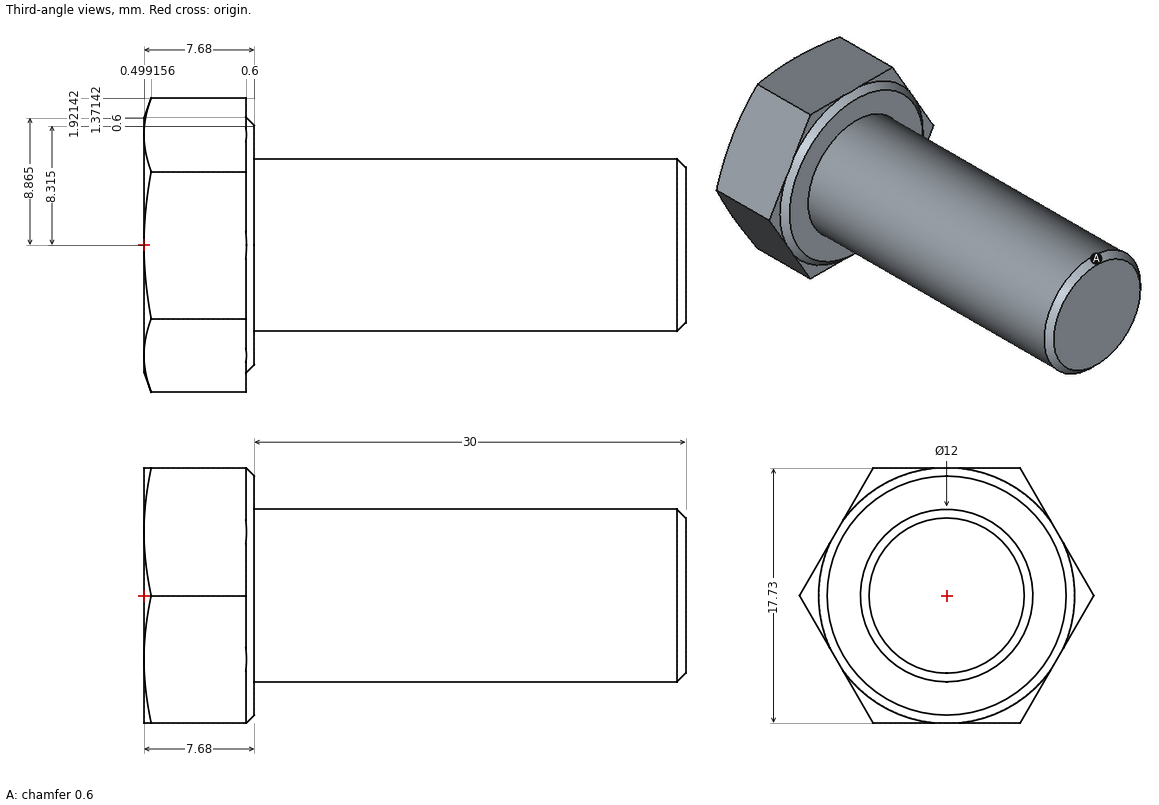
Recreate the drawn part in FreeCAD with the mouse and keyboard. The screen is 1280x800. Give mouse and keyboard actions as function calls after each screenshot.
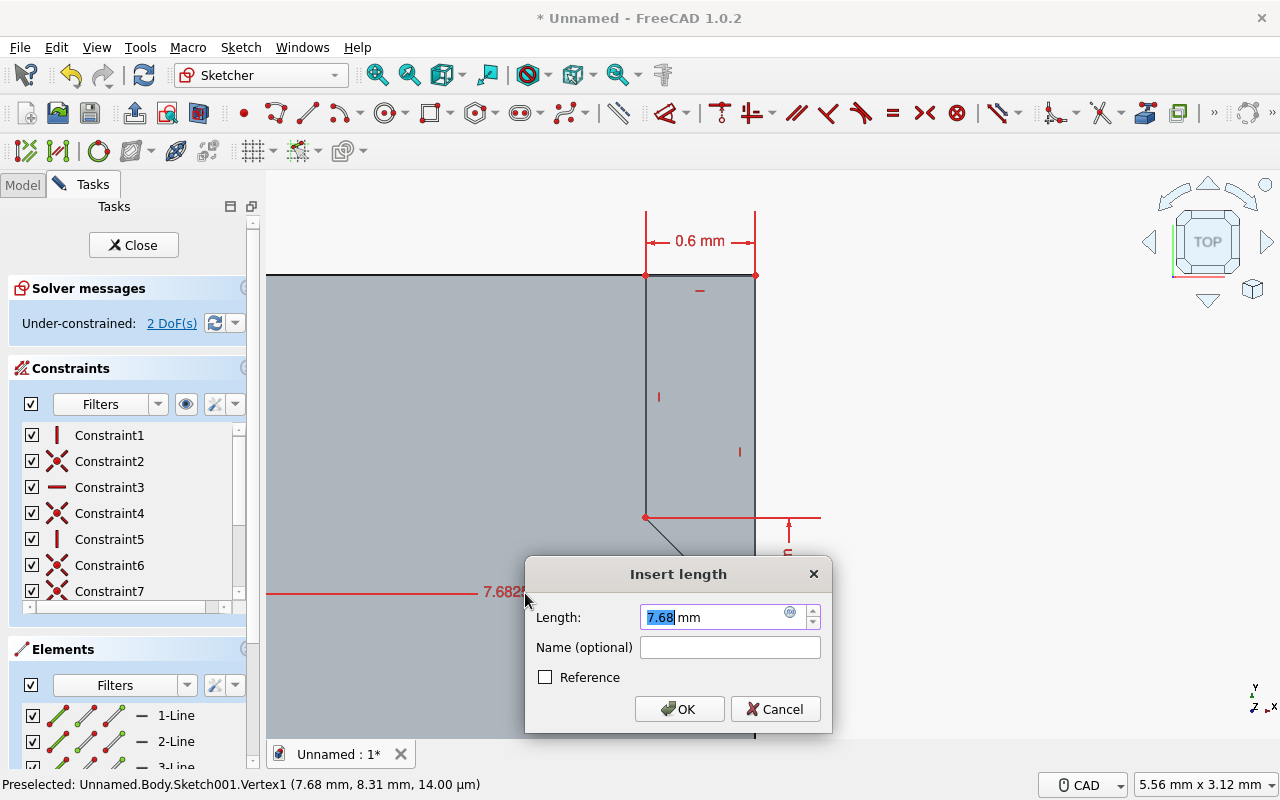
text(7.68)
key(Return)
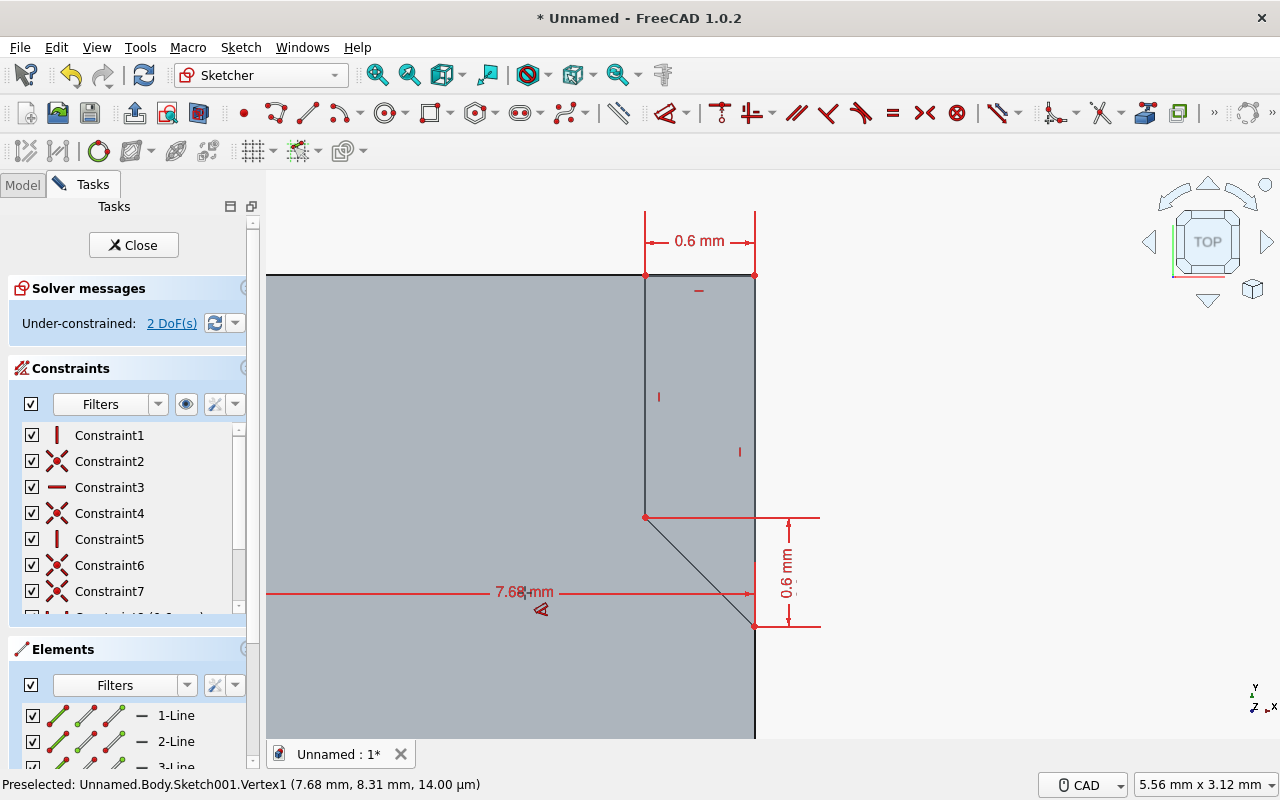
click(755, 627)
click(789, 669)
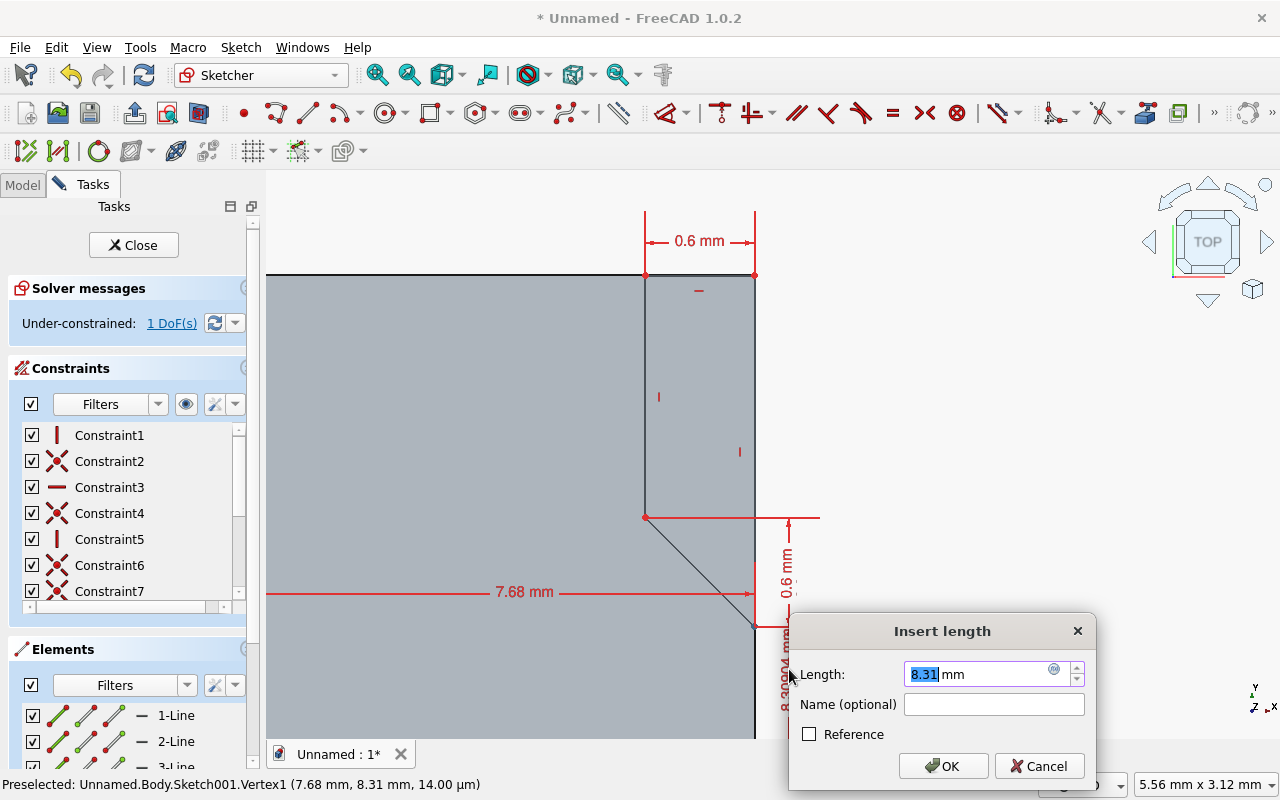
text(8.315)
key(Return)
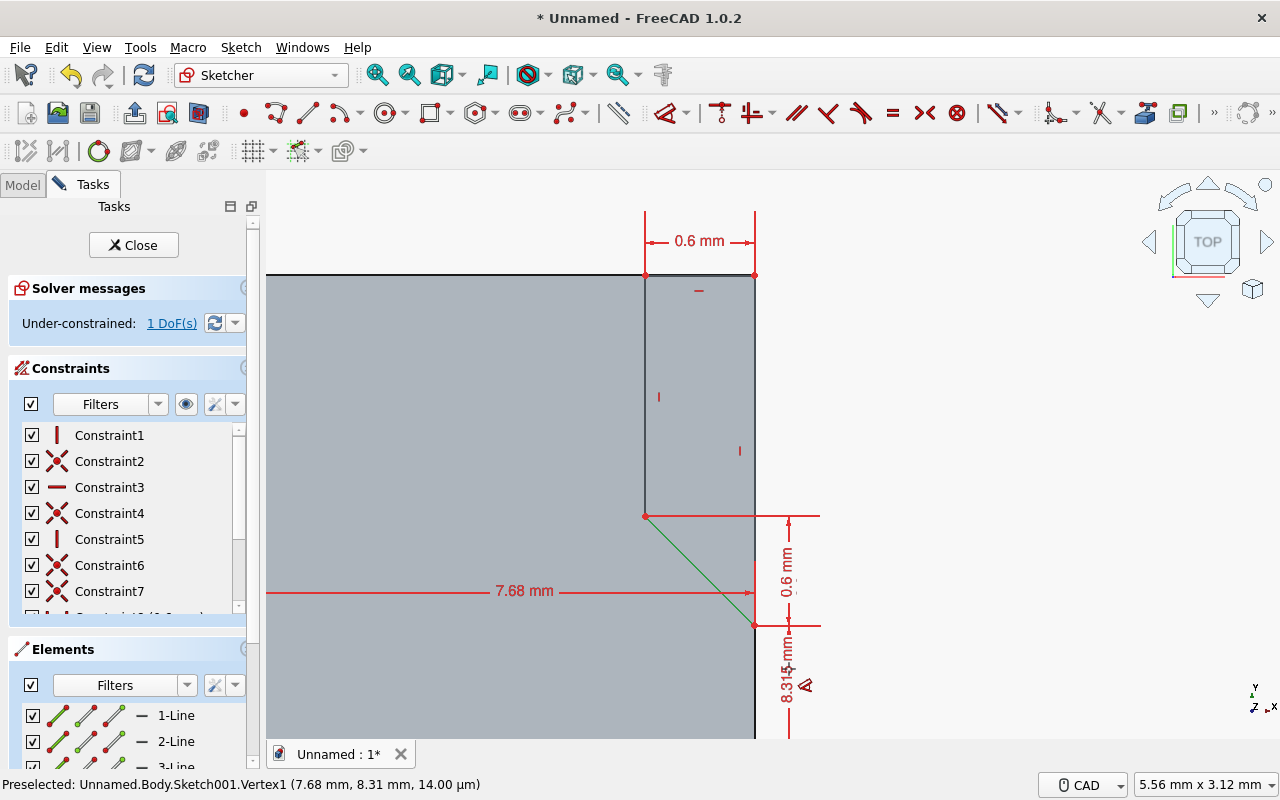
click(755, 521)
click(789, 451)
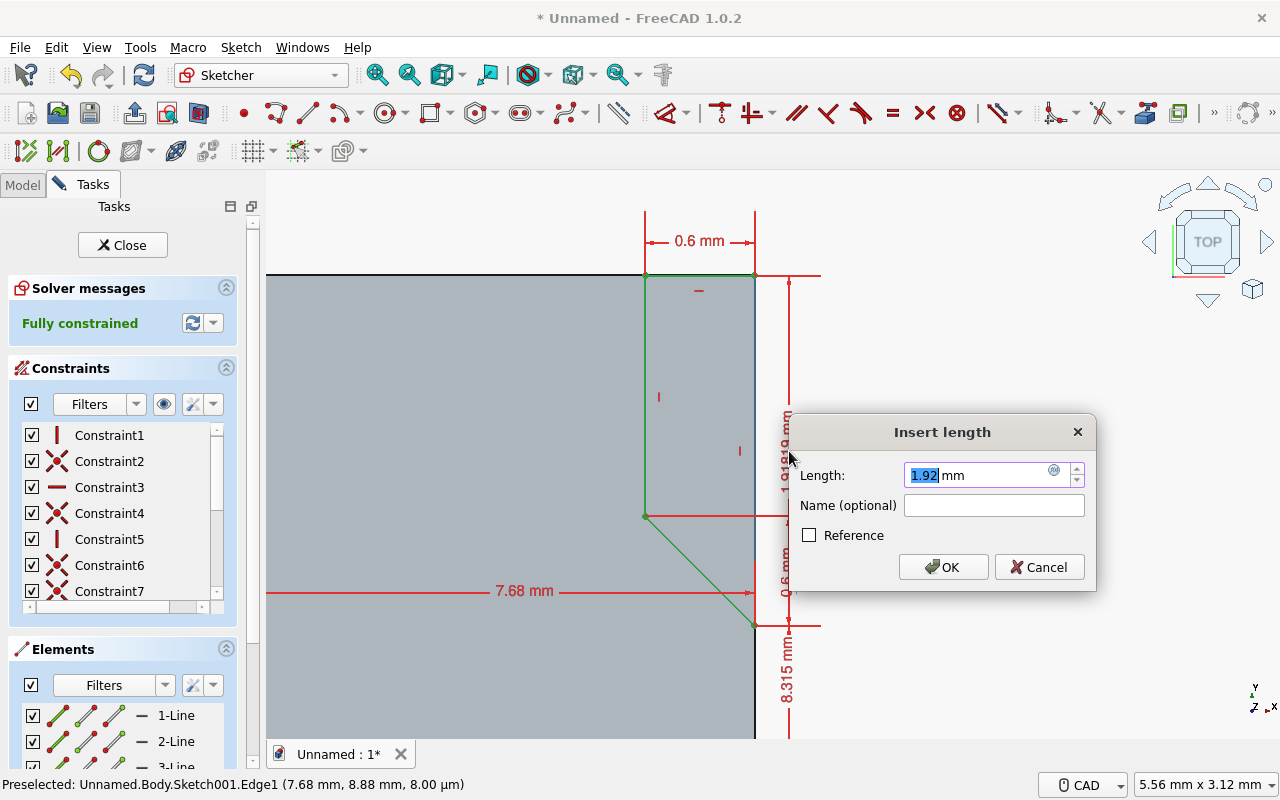
text(1.92142)
key(Return)
key(Escape)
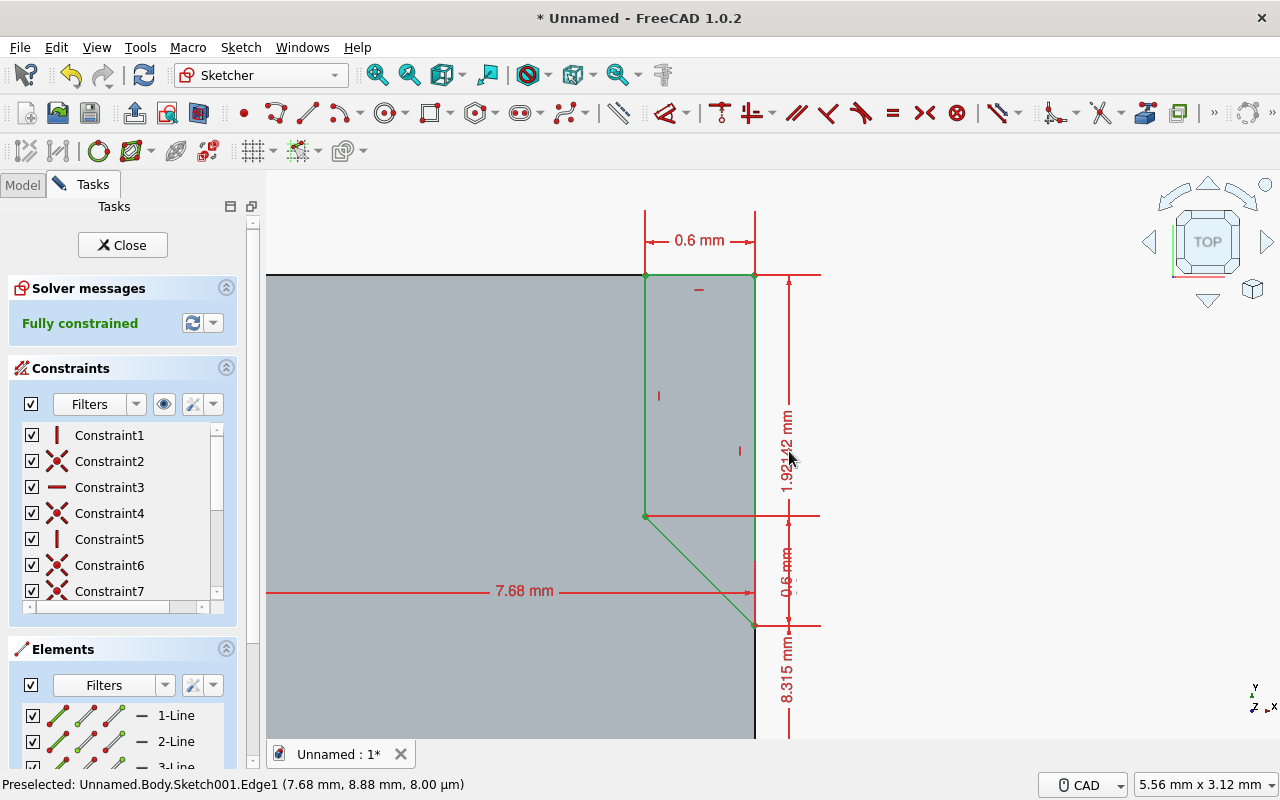
click(123, 245)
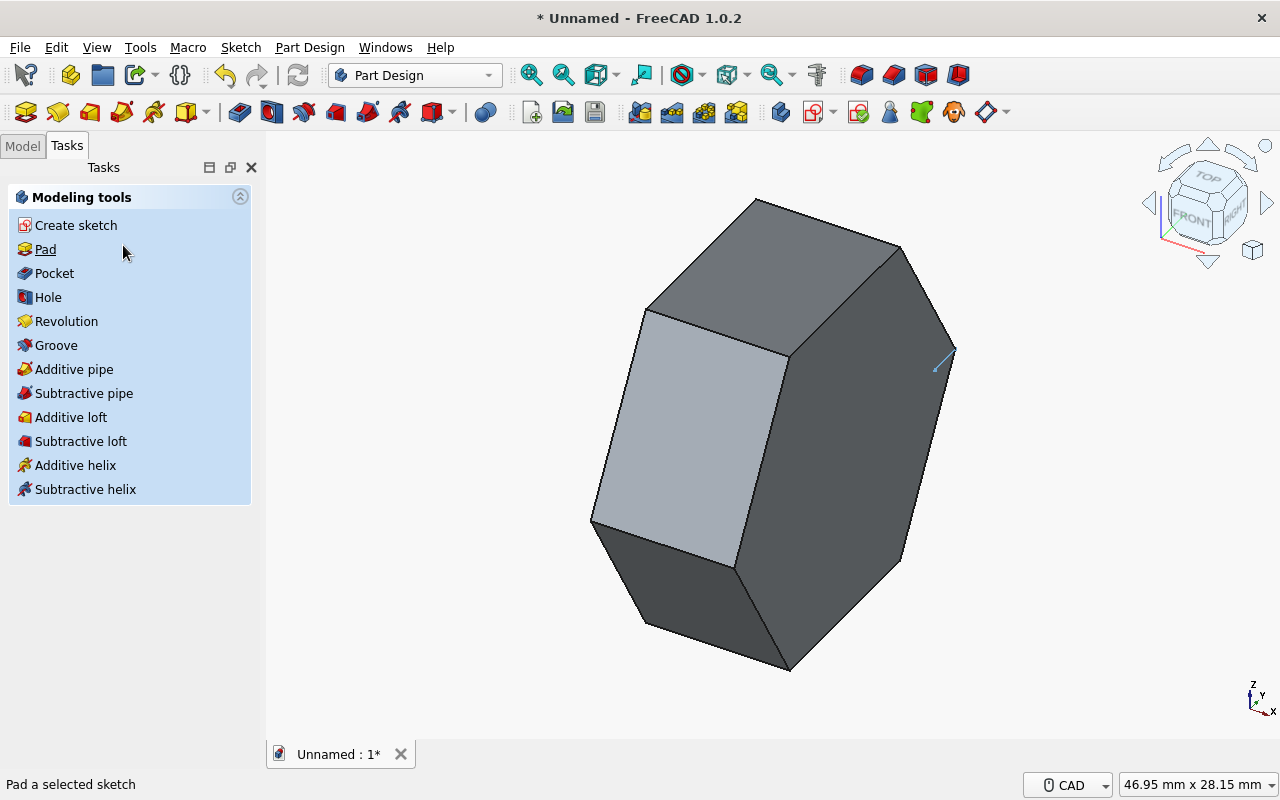
click(304, 112)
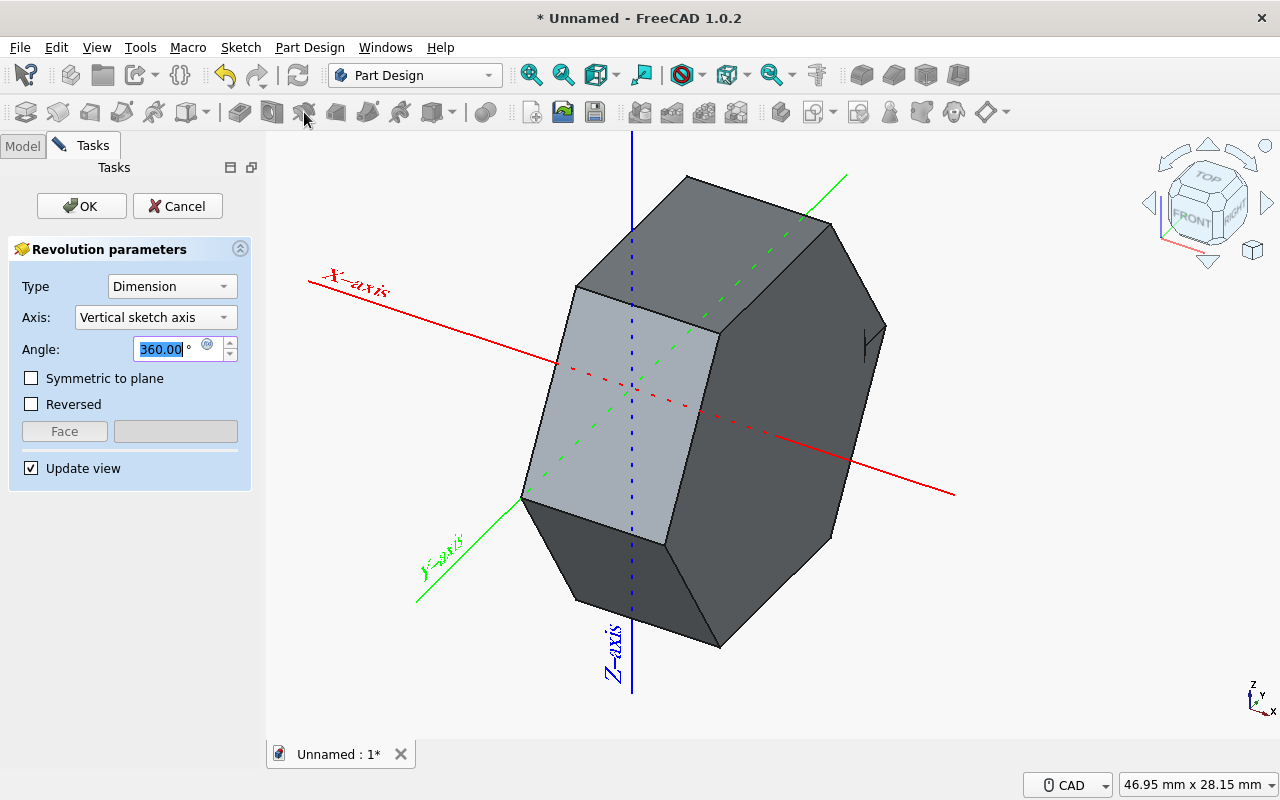
click(156, 318)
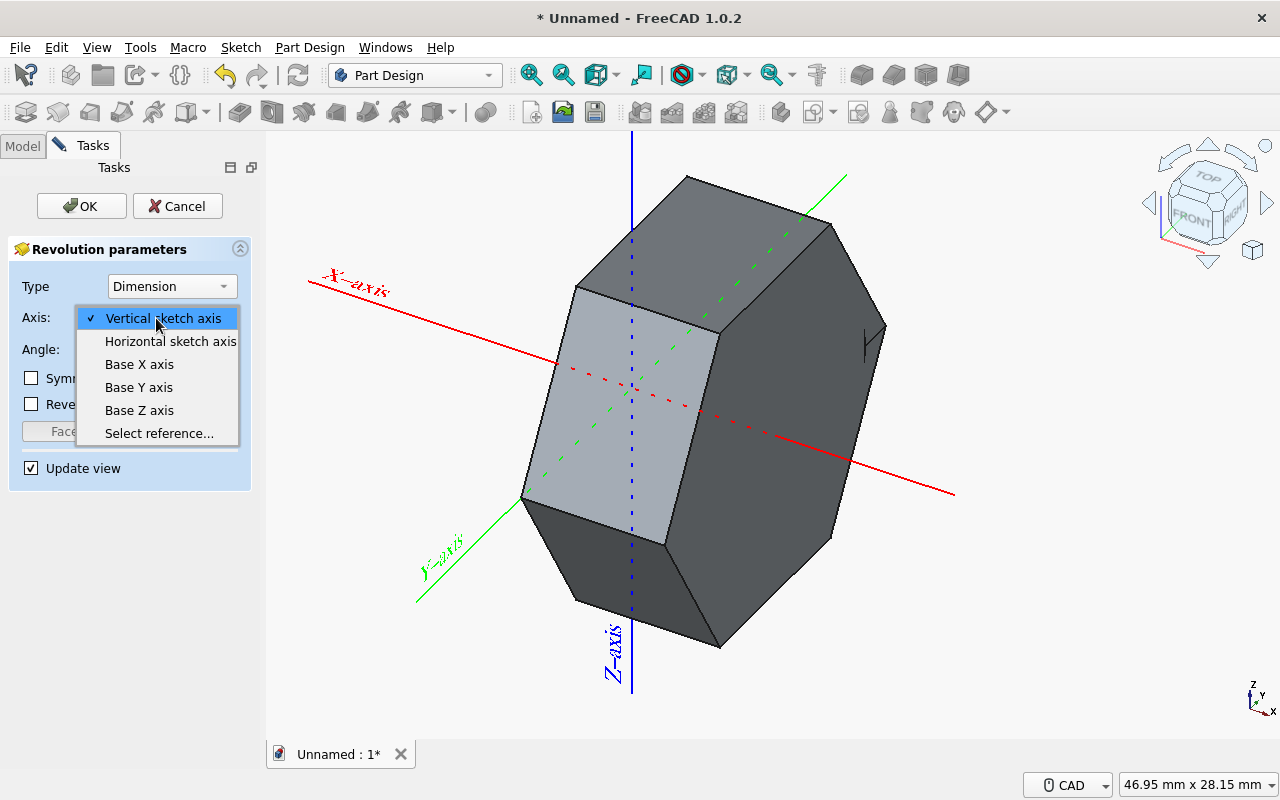
click(156, 342)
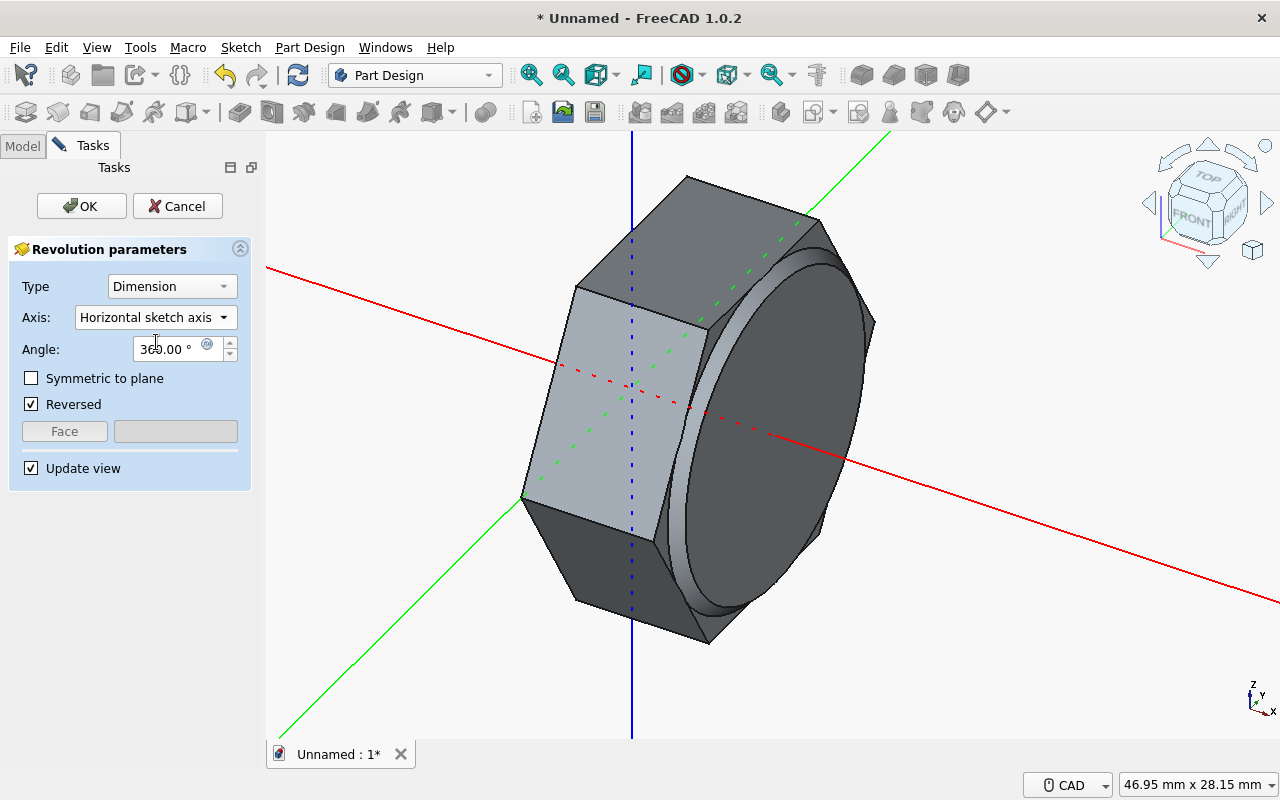
click(82, 206)